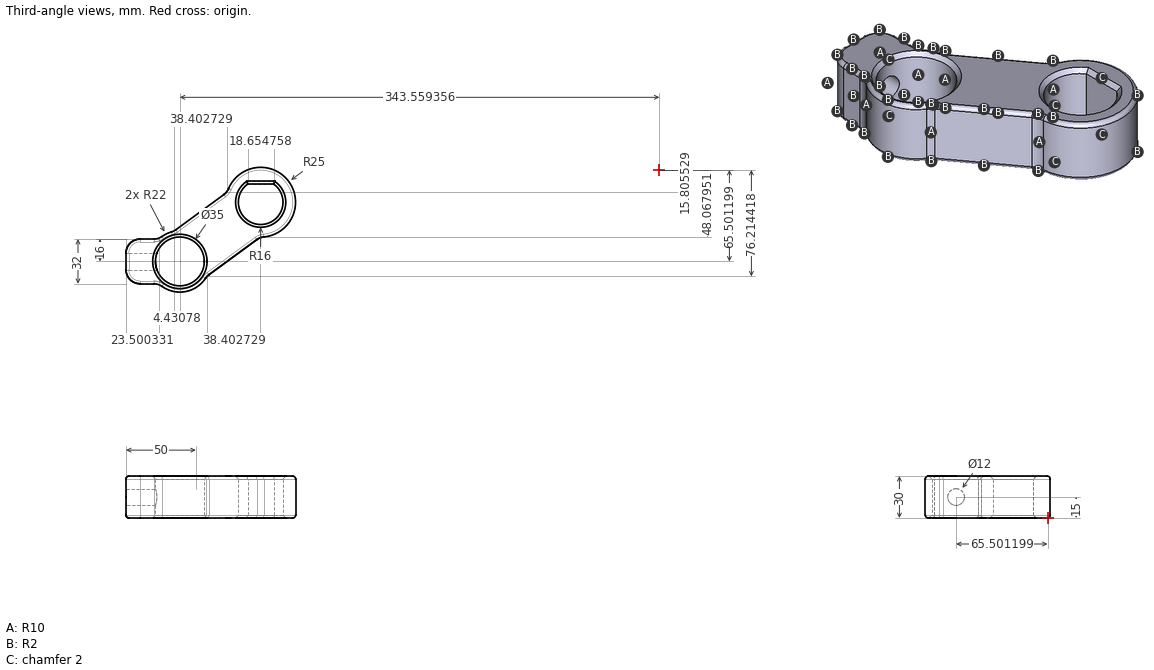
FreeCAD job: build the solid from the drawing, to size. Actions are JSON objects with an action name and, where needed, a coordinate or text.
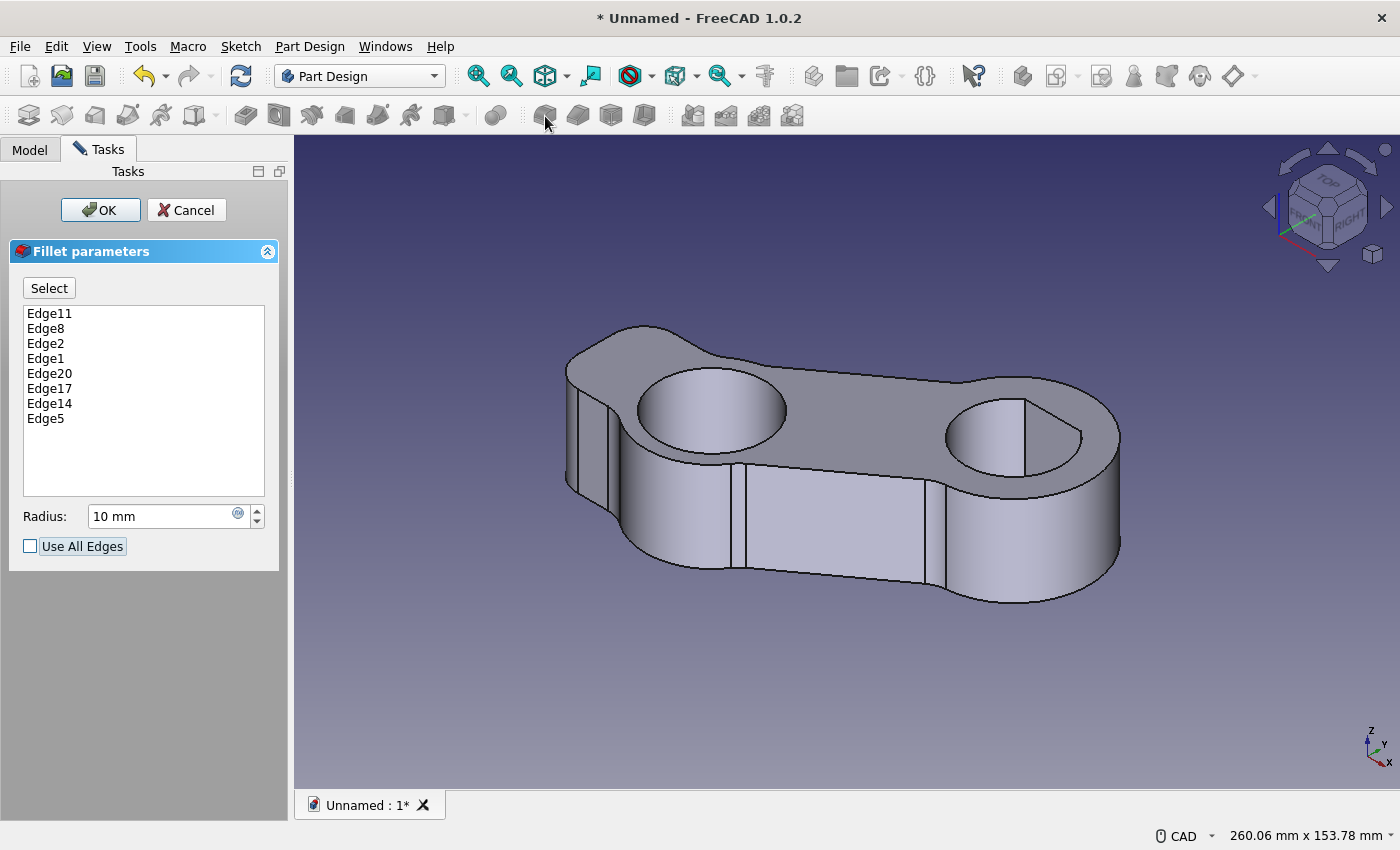
{"action": "left_click", "coordinate": [101, 210]}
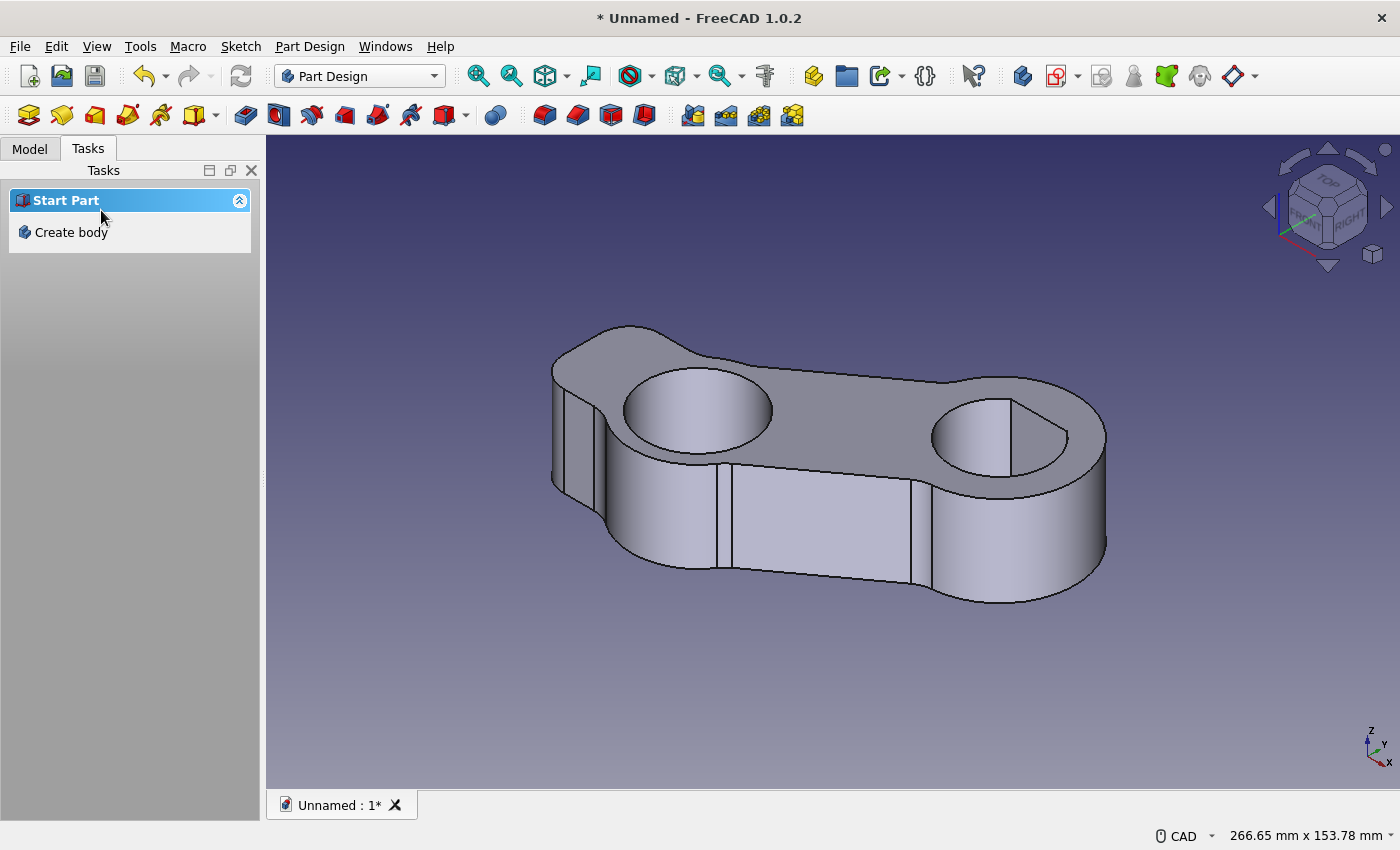
{"action": "left_click", "coordinate": [720, 357]}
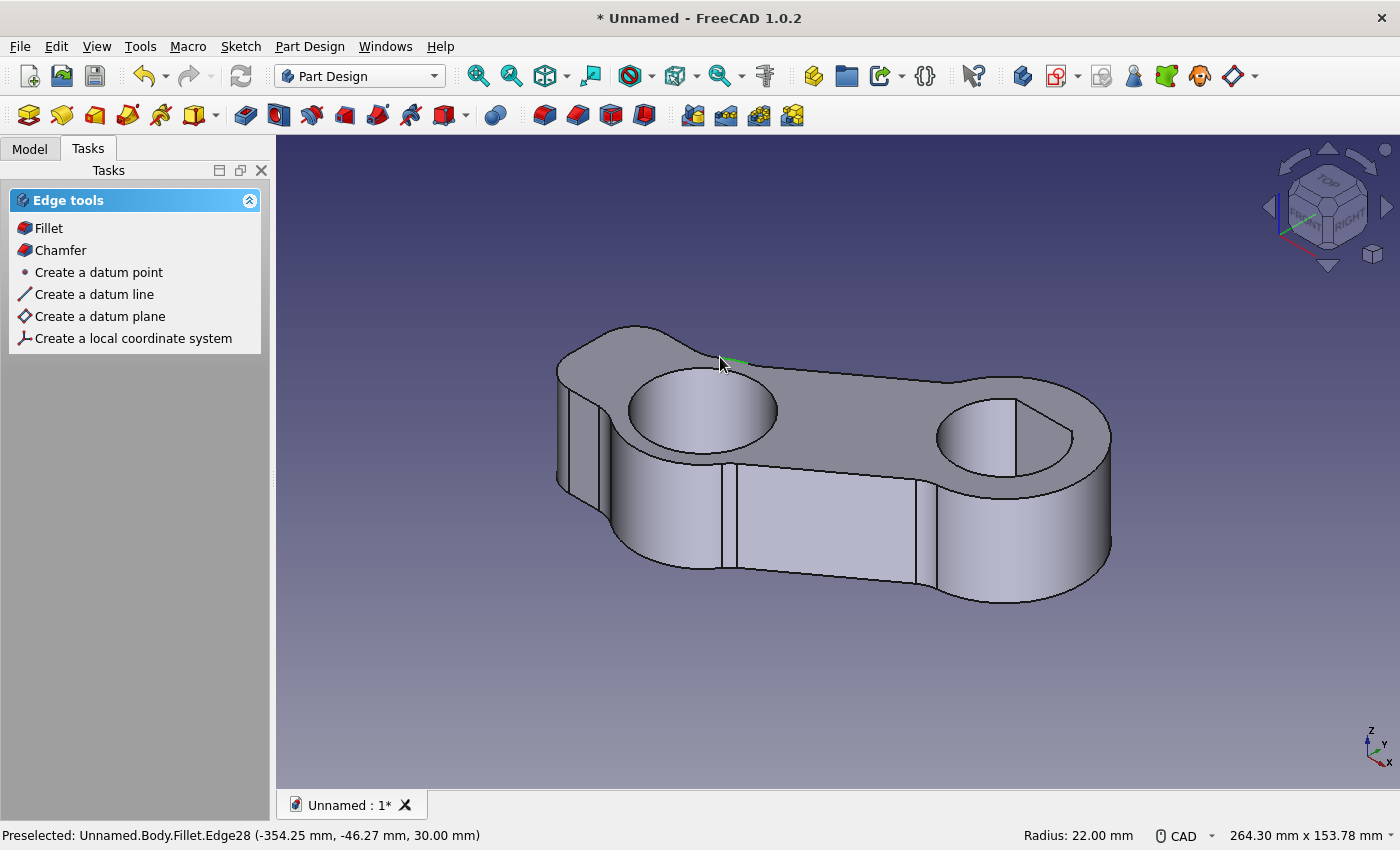
{"action": "left_click", "coordinate": [1110, 446], "text": "ctrl"}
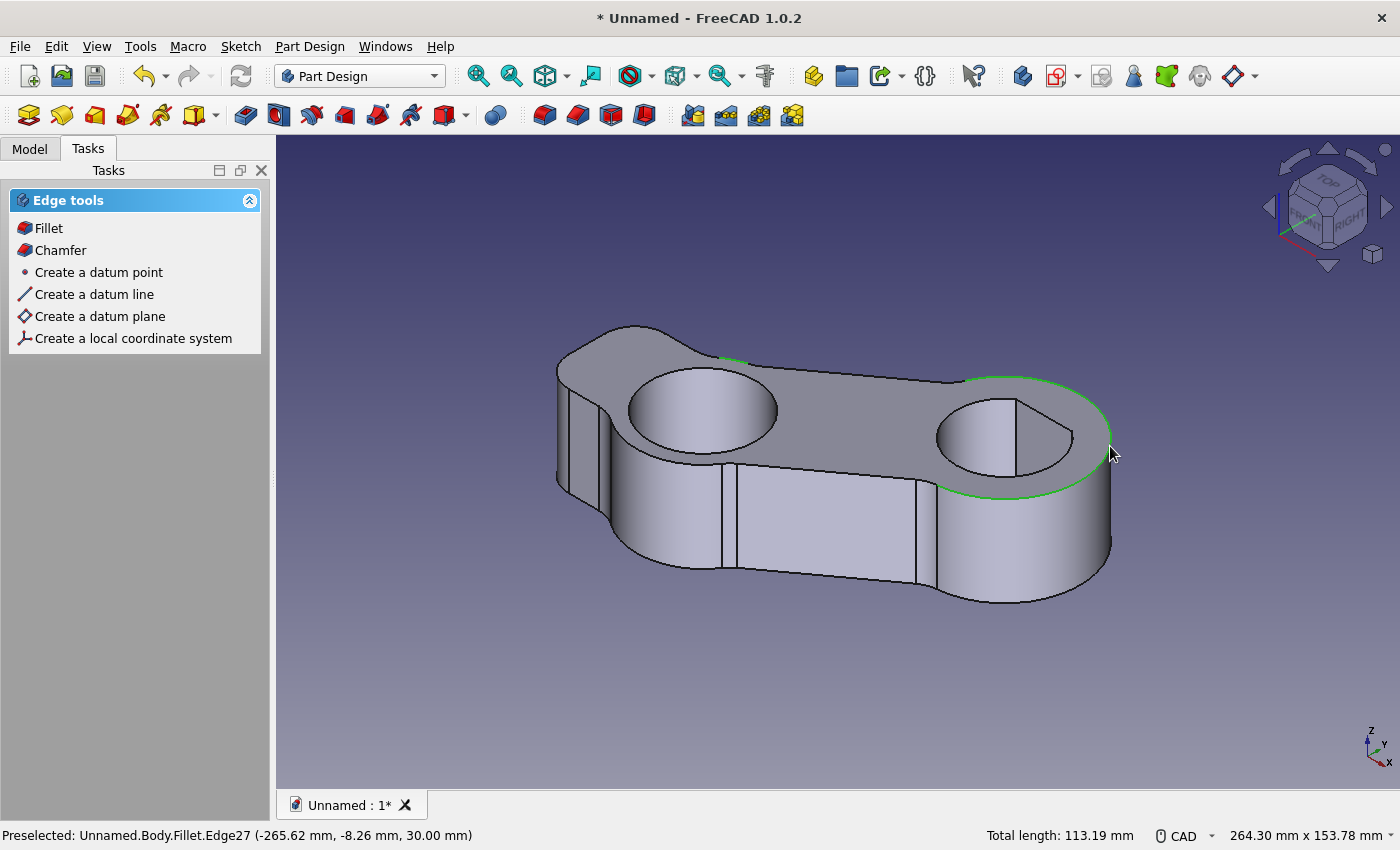
{"action": "left_click", "coordinate": [826, 471], "text": "ctrl"}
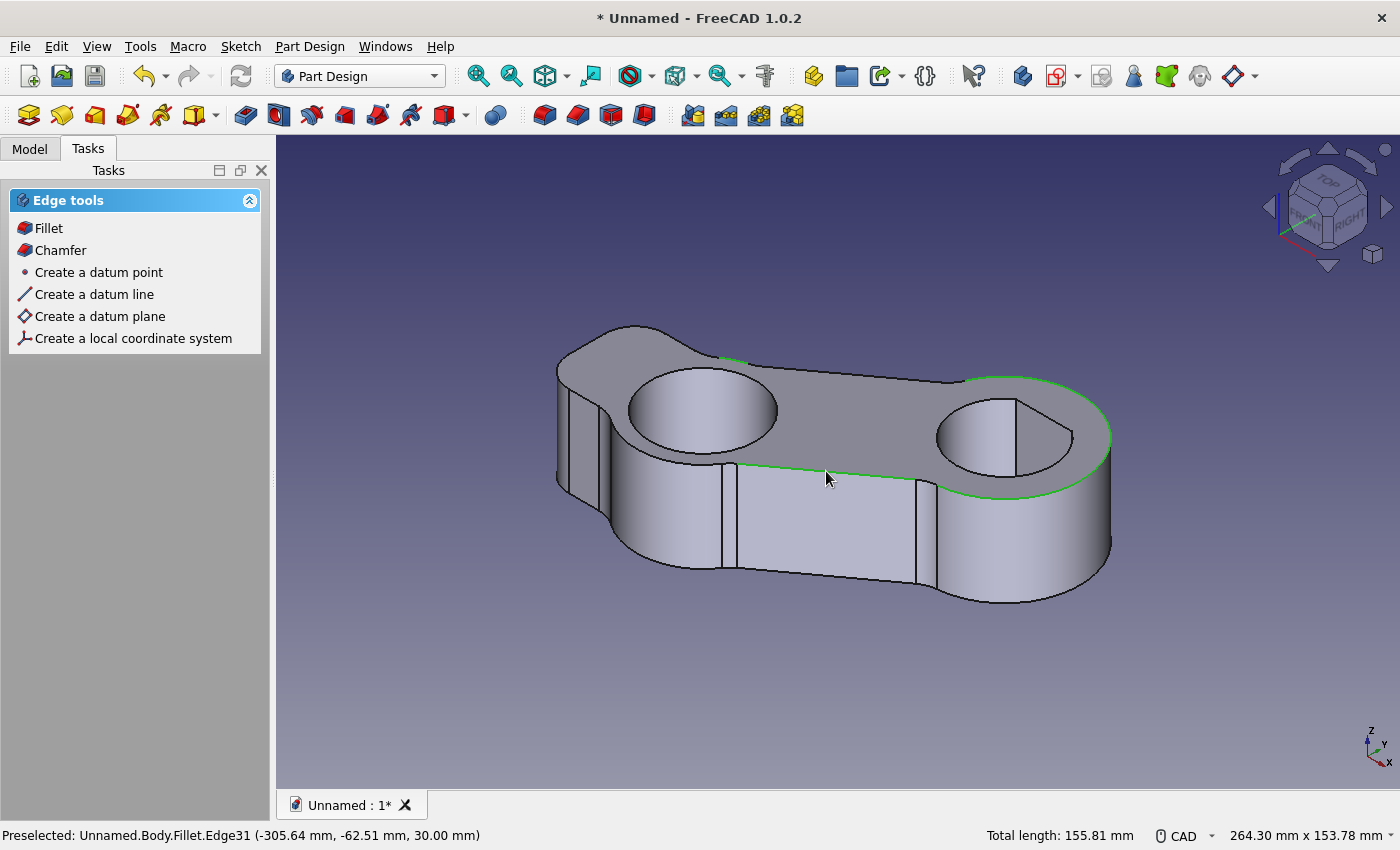
{"action": "left_click", "coordinate": [650, 454], "text": "ctrl"}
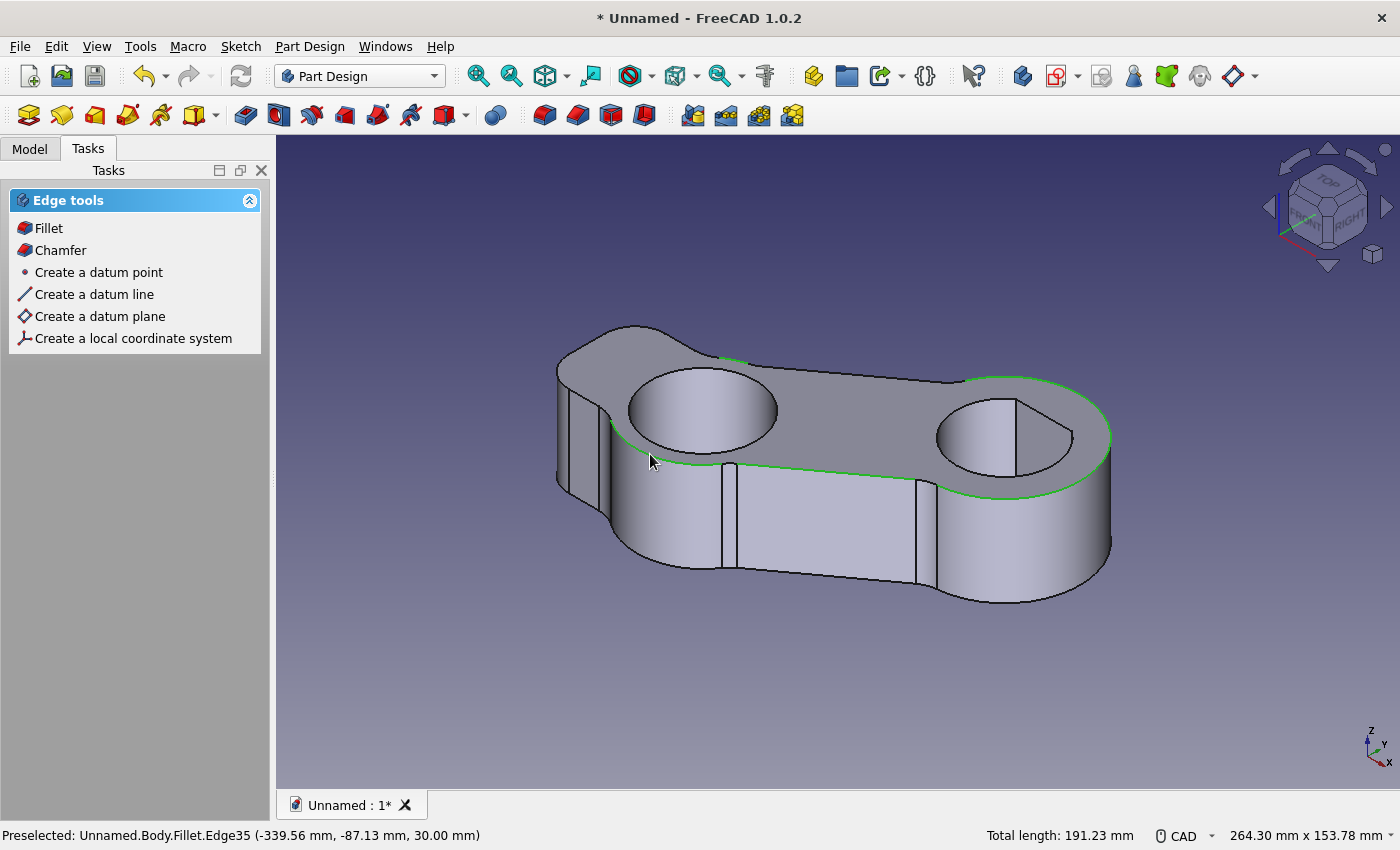
{"action": "left_click", "coordinate": [584, 397], "text": "ctrl"}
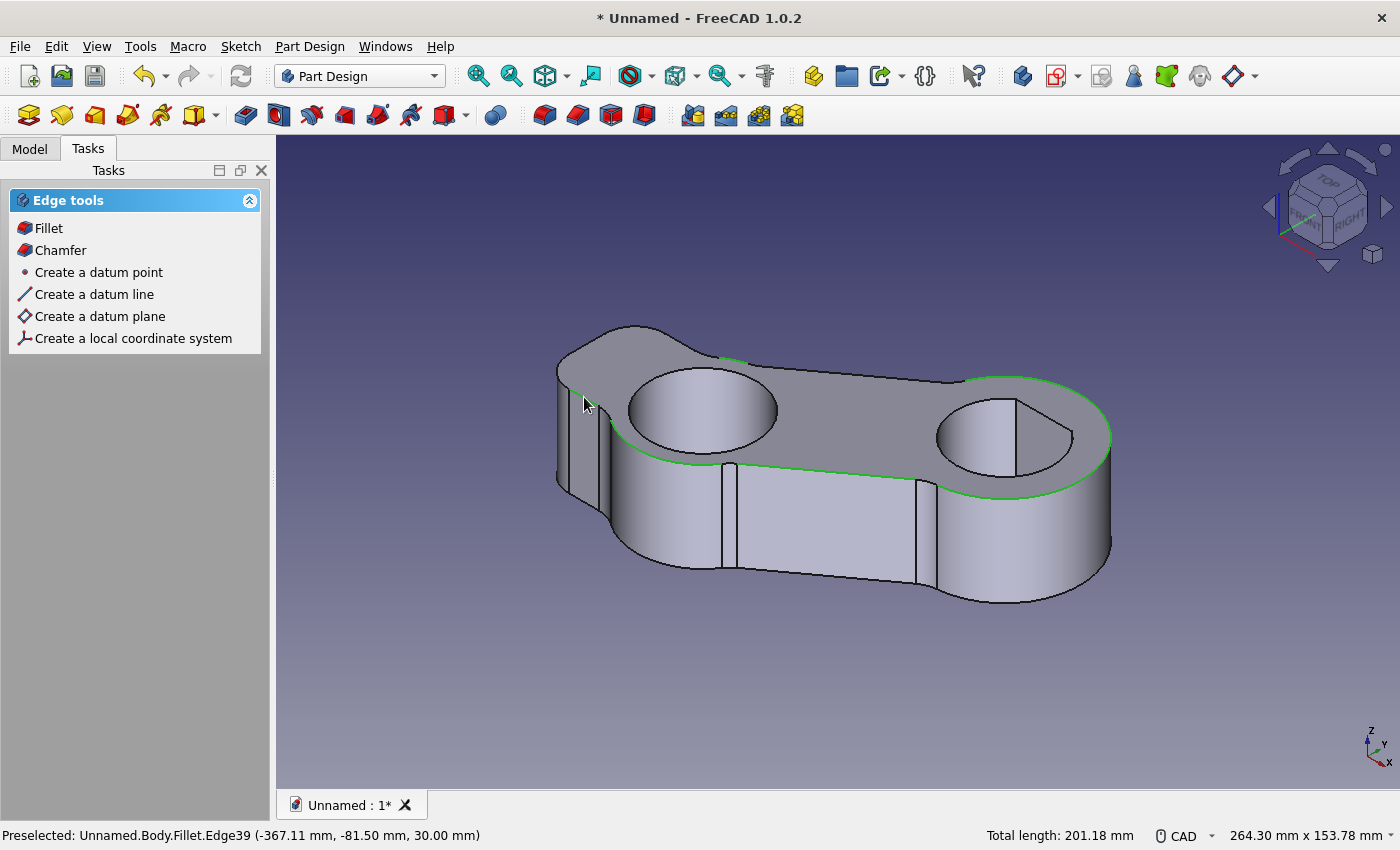
{"action": "left_click", "coordinate": [561, 486], "text": "ctrl"}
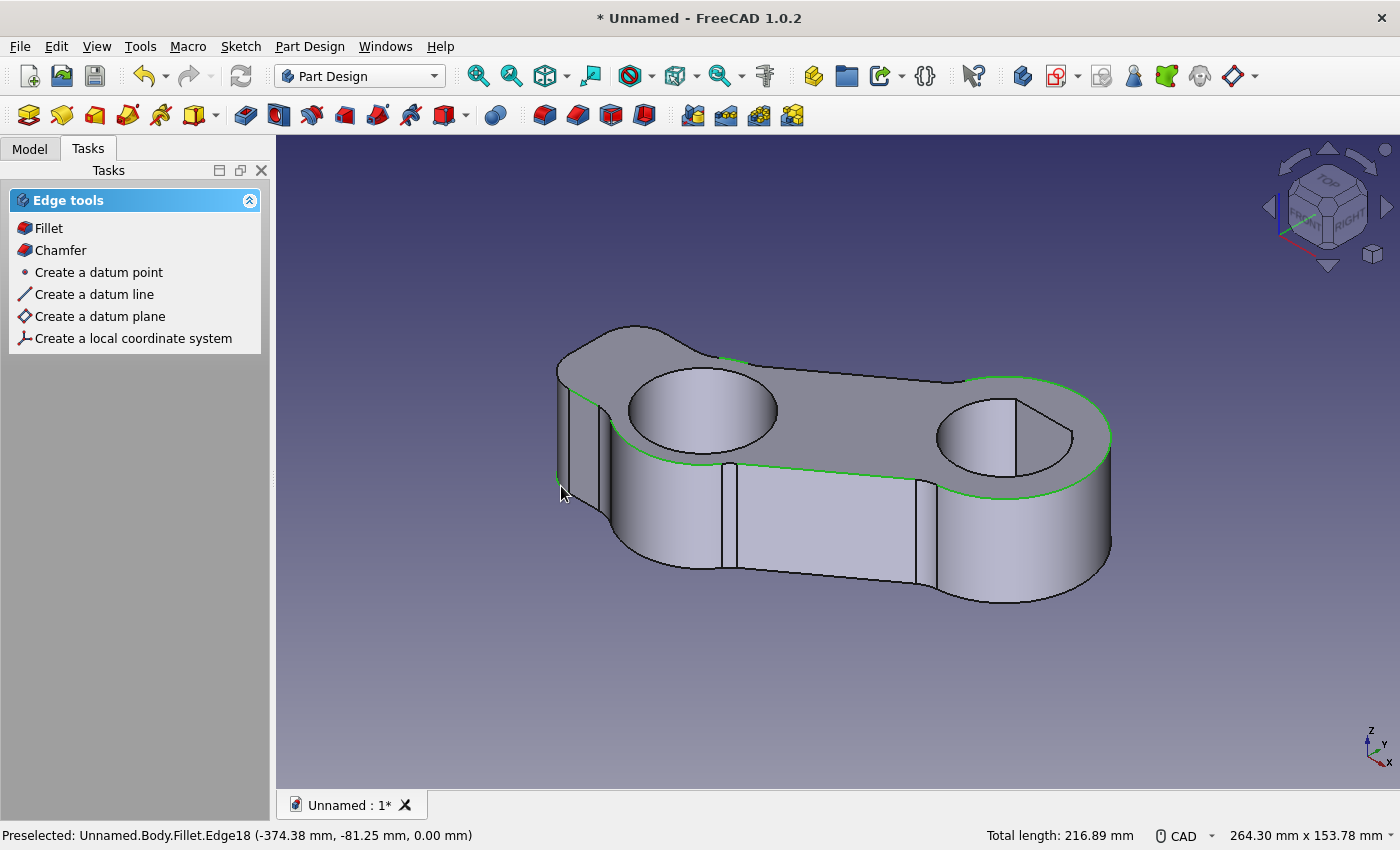
{"action": "left_click", "coordinate": [557, 367], "text": "ctrl"}